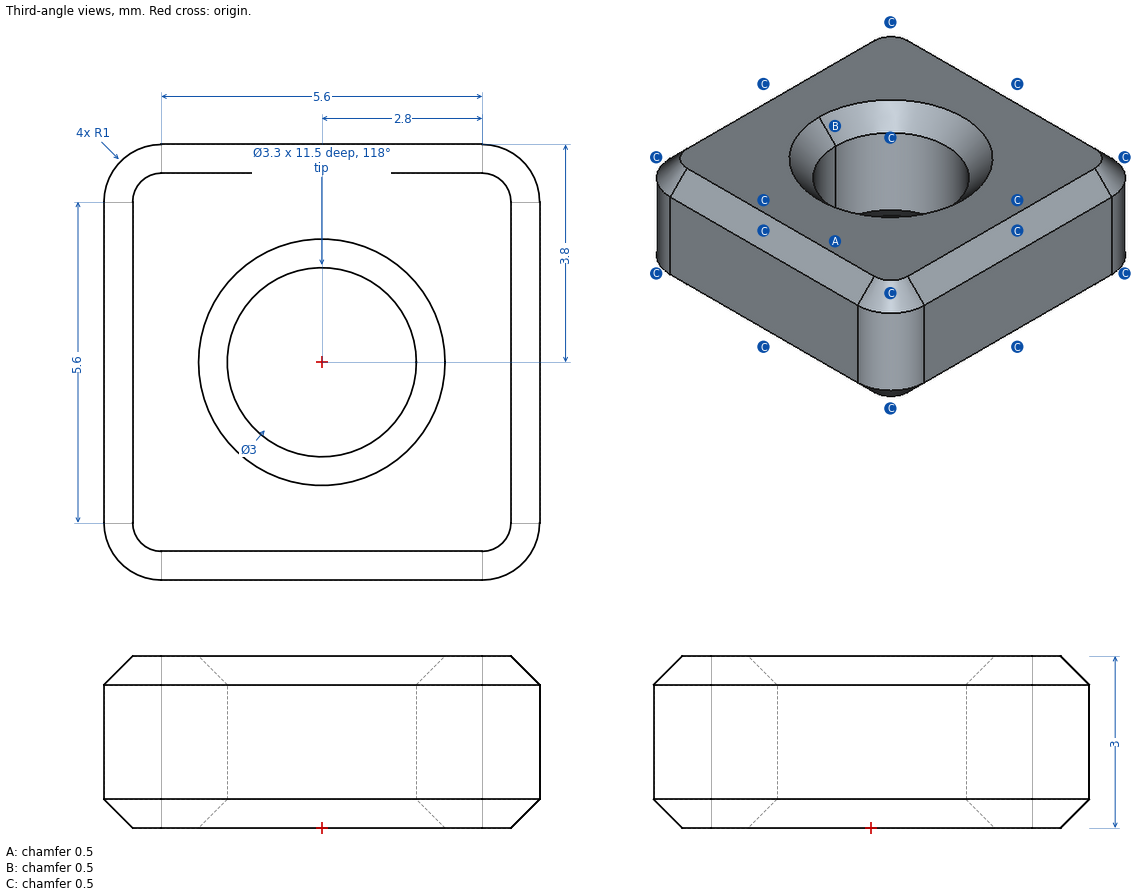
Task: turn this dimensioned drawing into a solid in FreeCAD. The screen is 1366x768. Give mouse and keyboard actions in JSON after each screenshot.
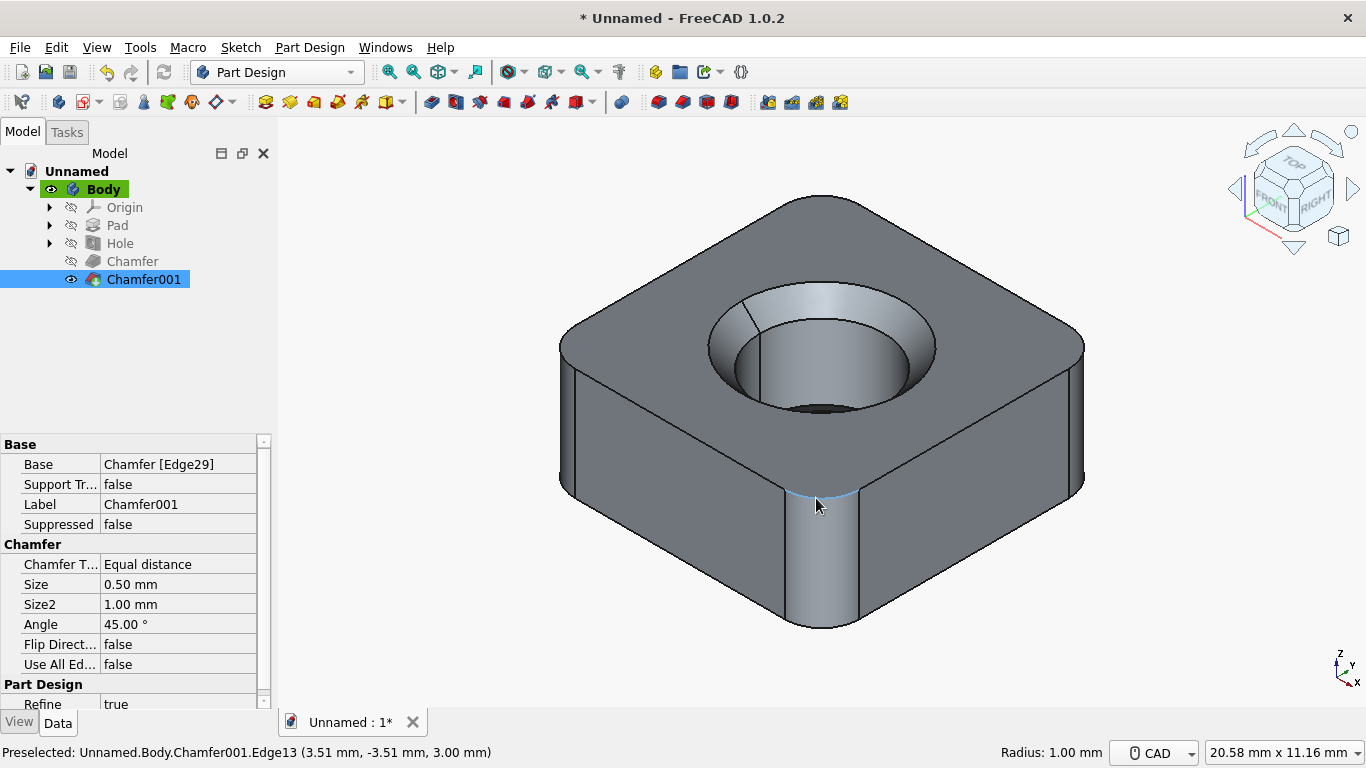
{"action": "left_click", "coordinate": [562, 485], "text": "ctrl"}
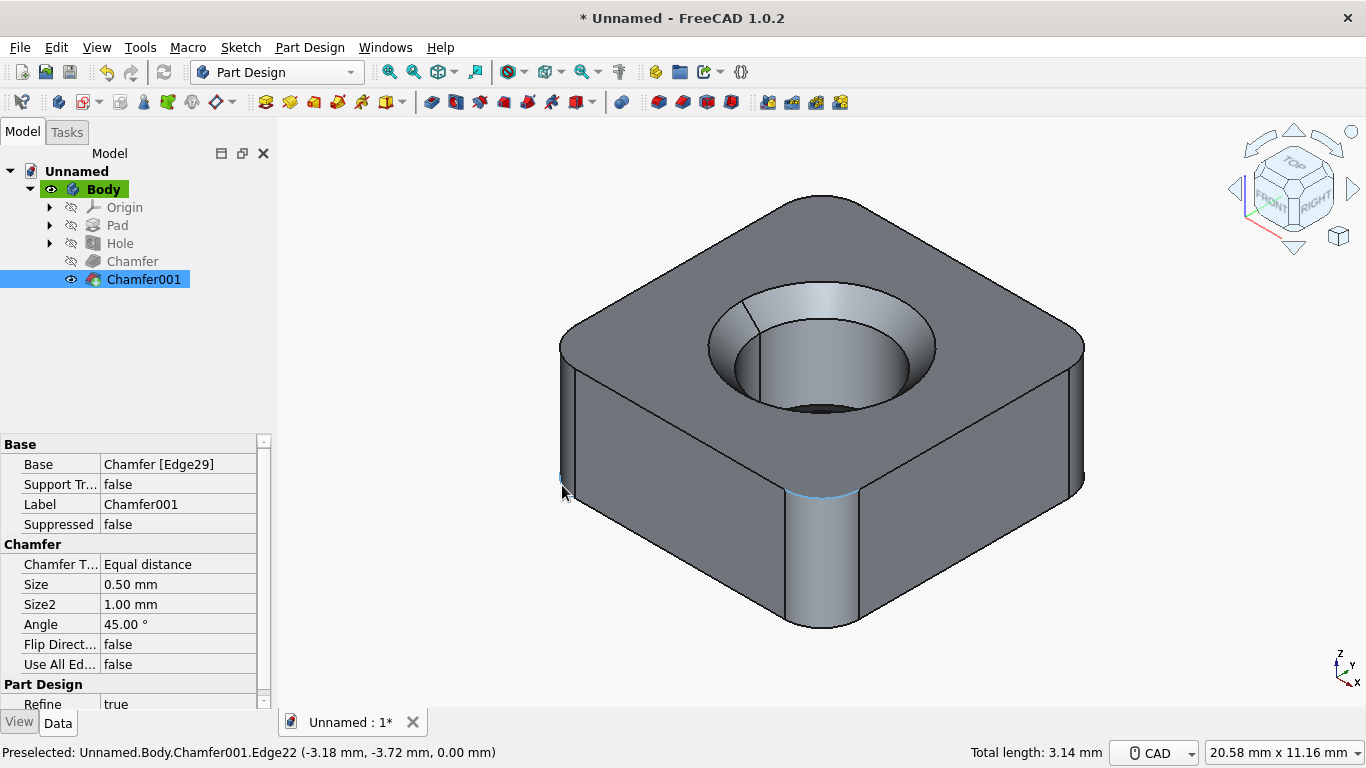
{"action": "left_click", "coordinate": [964, 428], "text": "ctrl"}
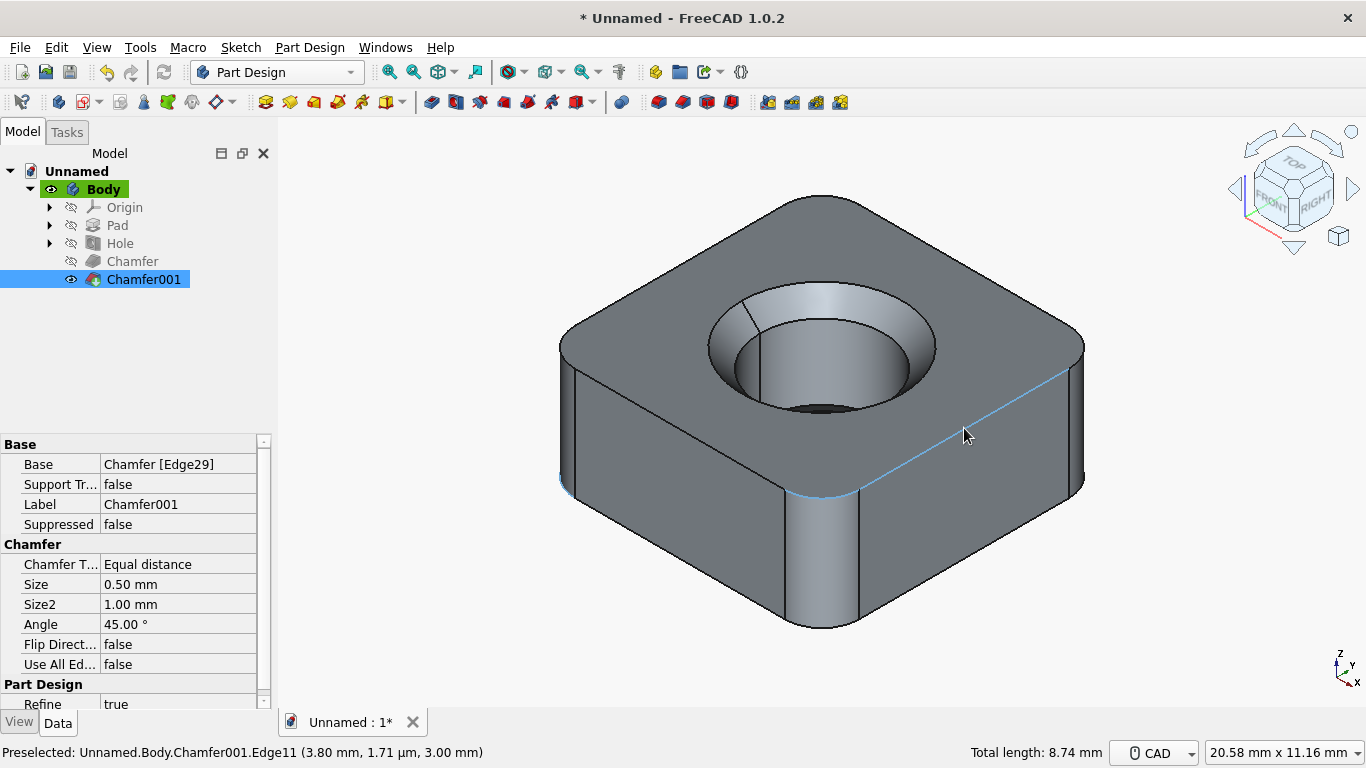
{"action": "left_click", "coordinate": [1084, 346], "text": "ctrl"}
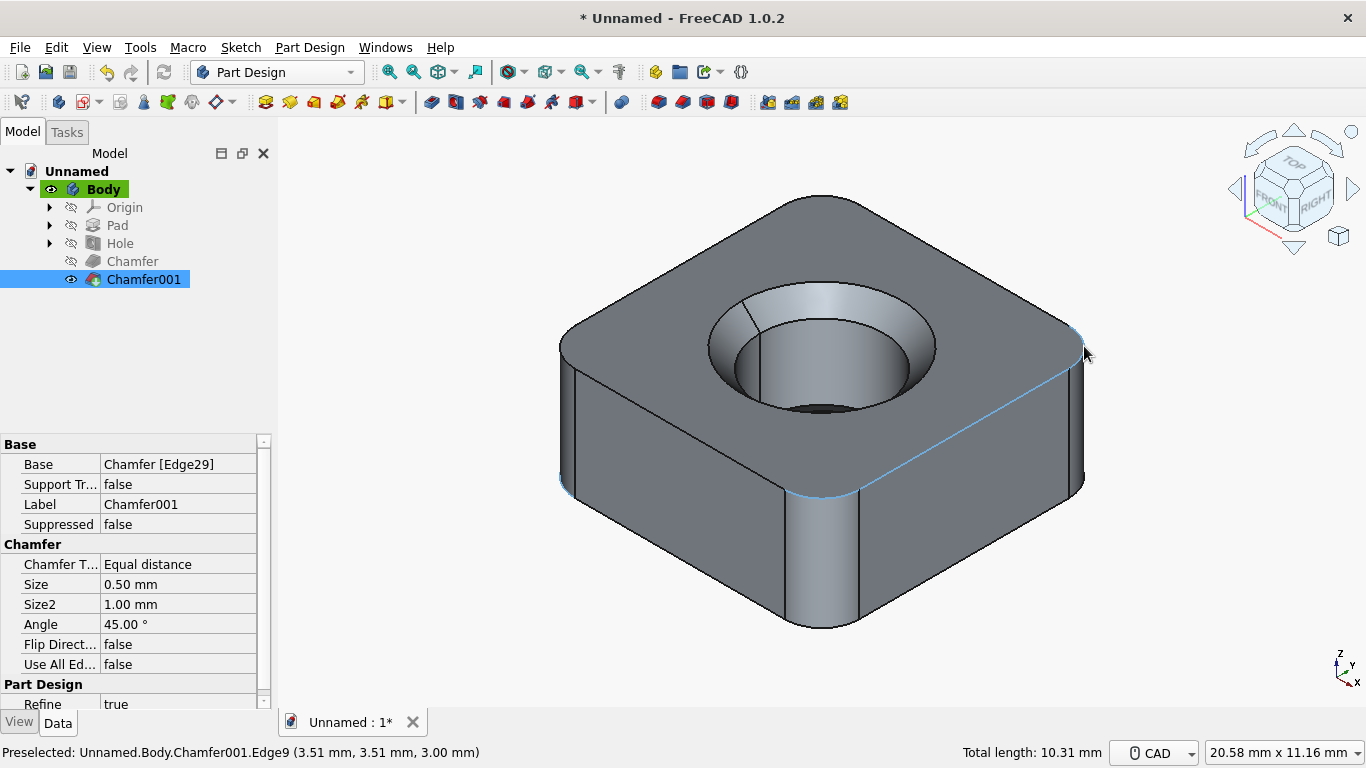
{"action": "left_click", "coordinate": [560, 346], "text": "ctrl"}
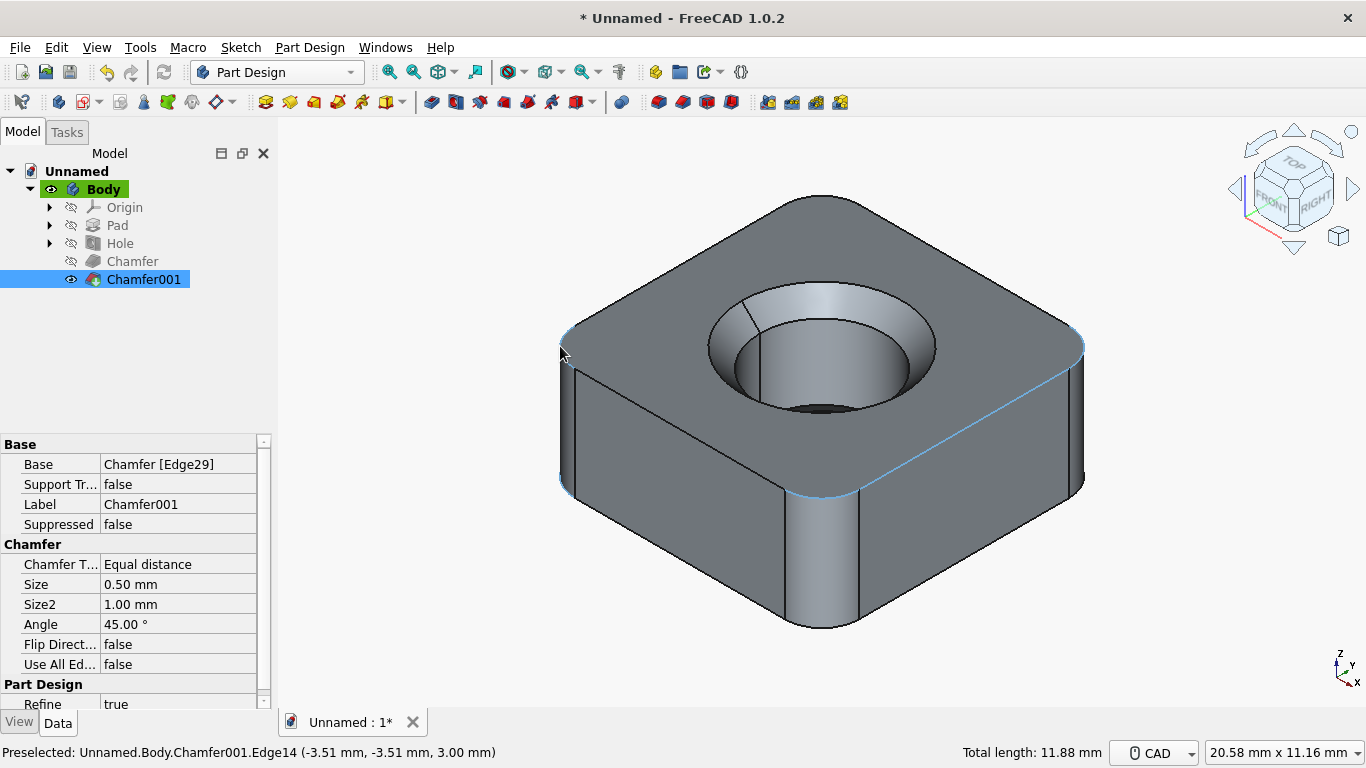
{"action": "left_click", "coordinate": [680, 428], "text": "ctrl"}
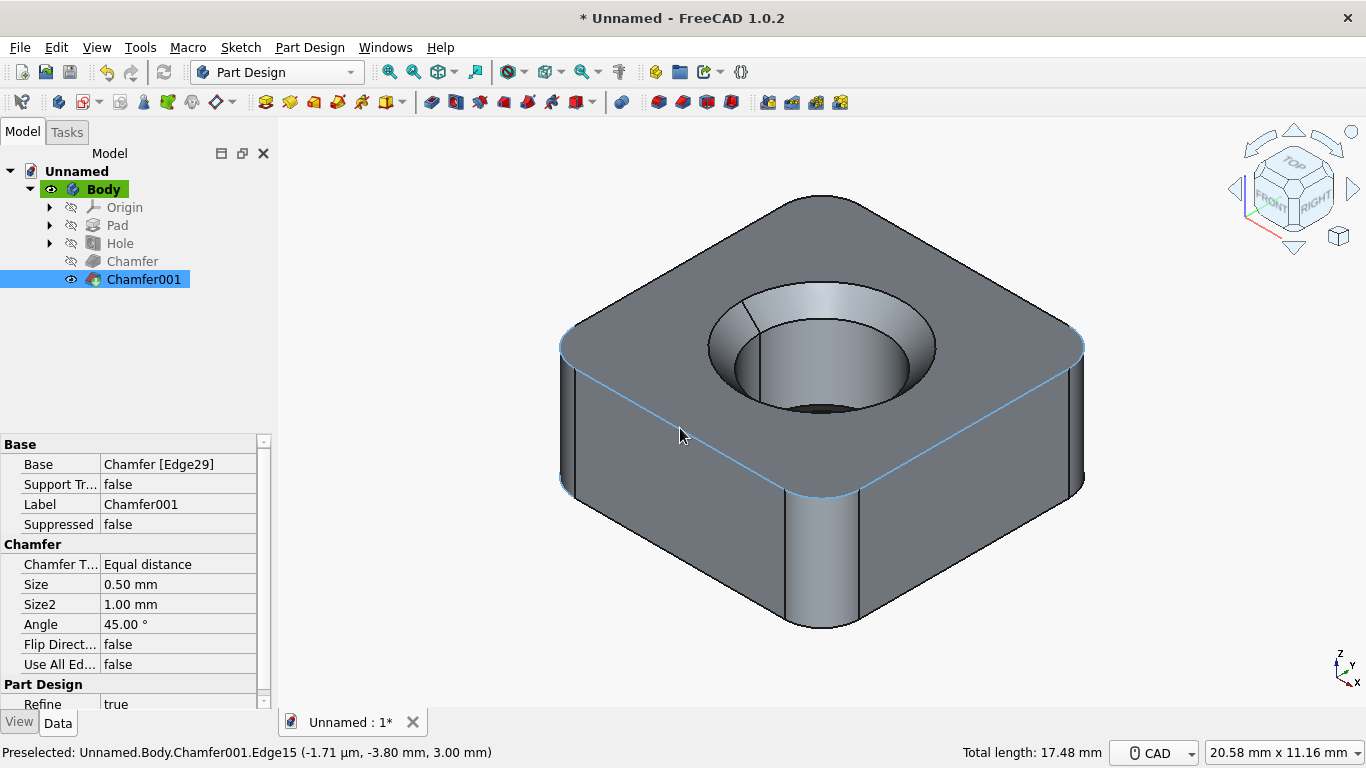
{"action": "left_click", "coordinate": [1082, 485], "text": "ctrl"}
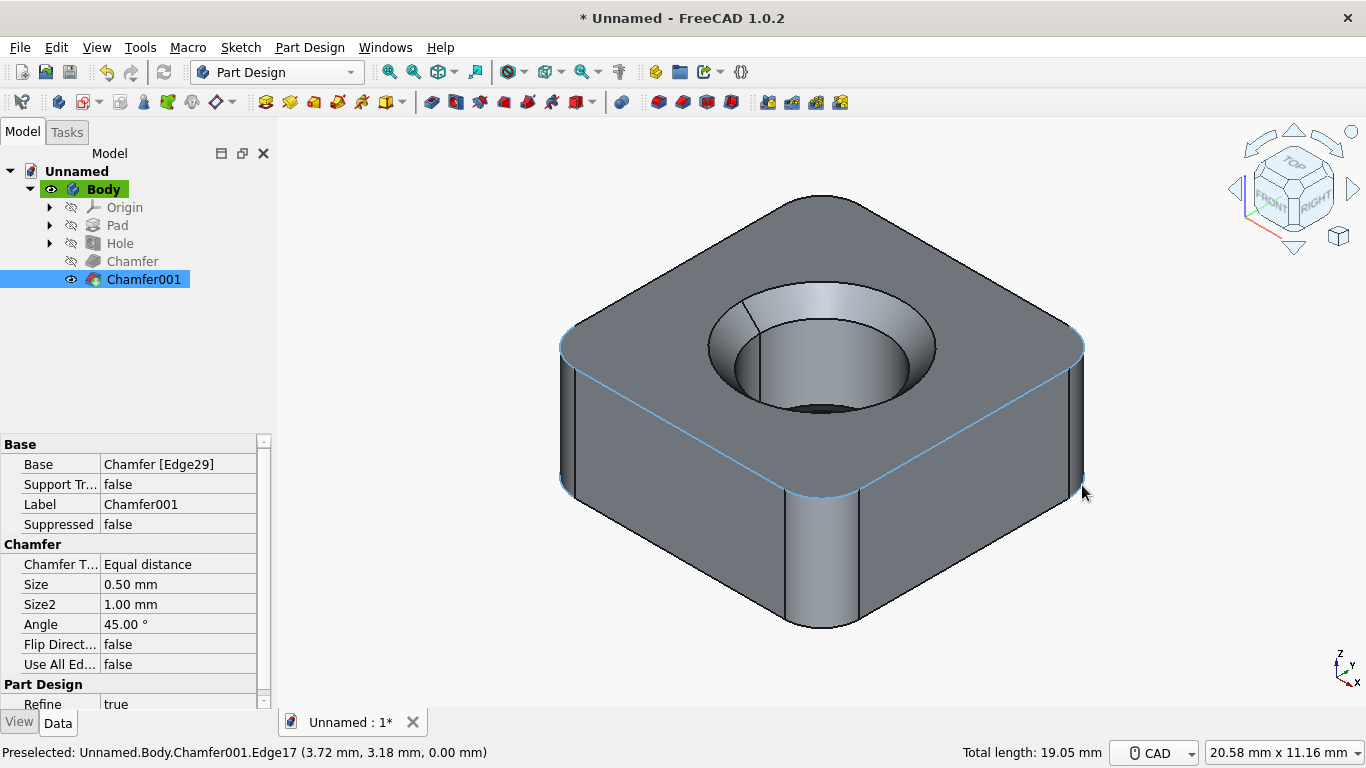
{"action": "key", "text": "2"}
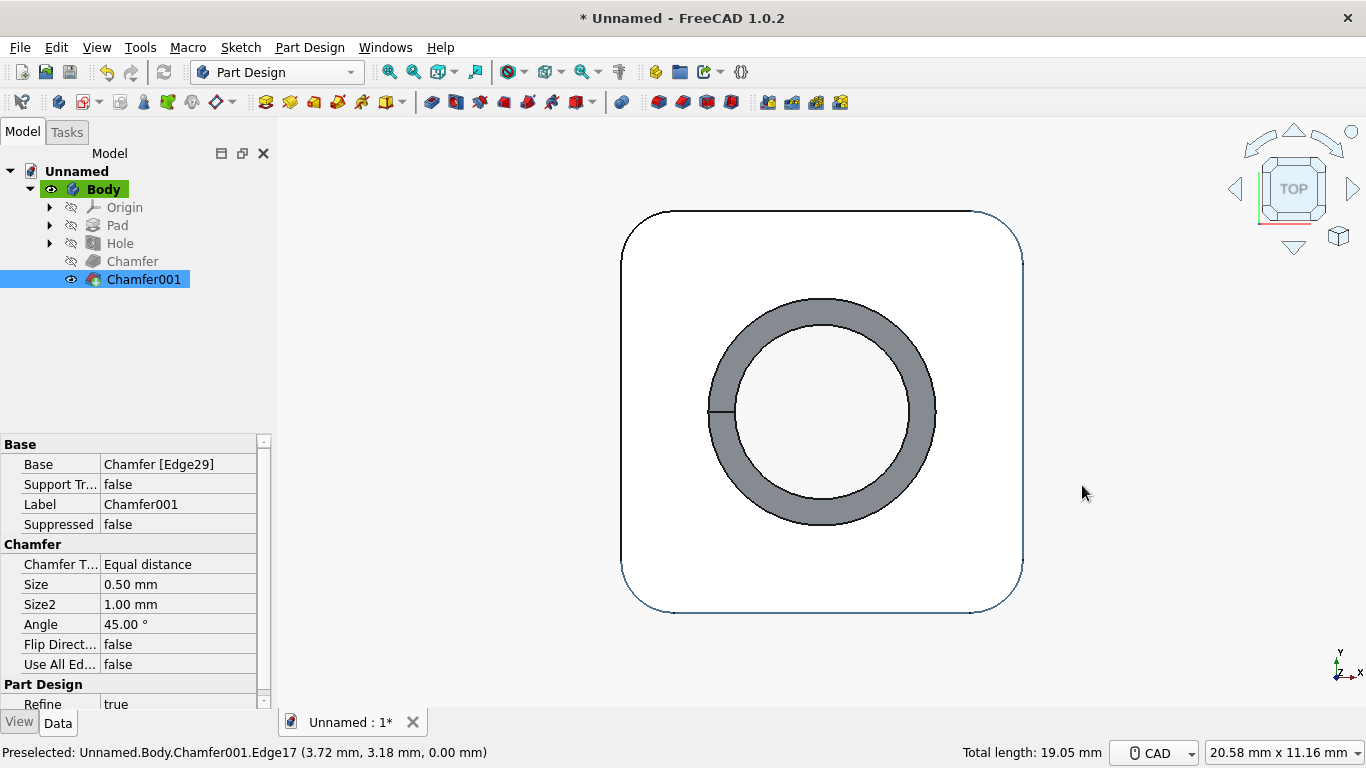
{"action": "left_click", "coordinate": [822, 210], "text": "ctrl"}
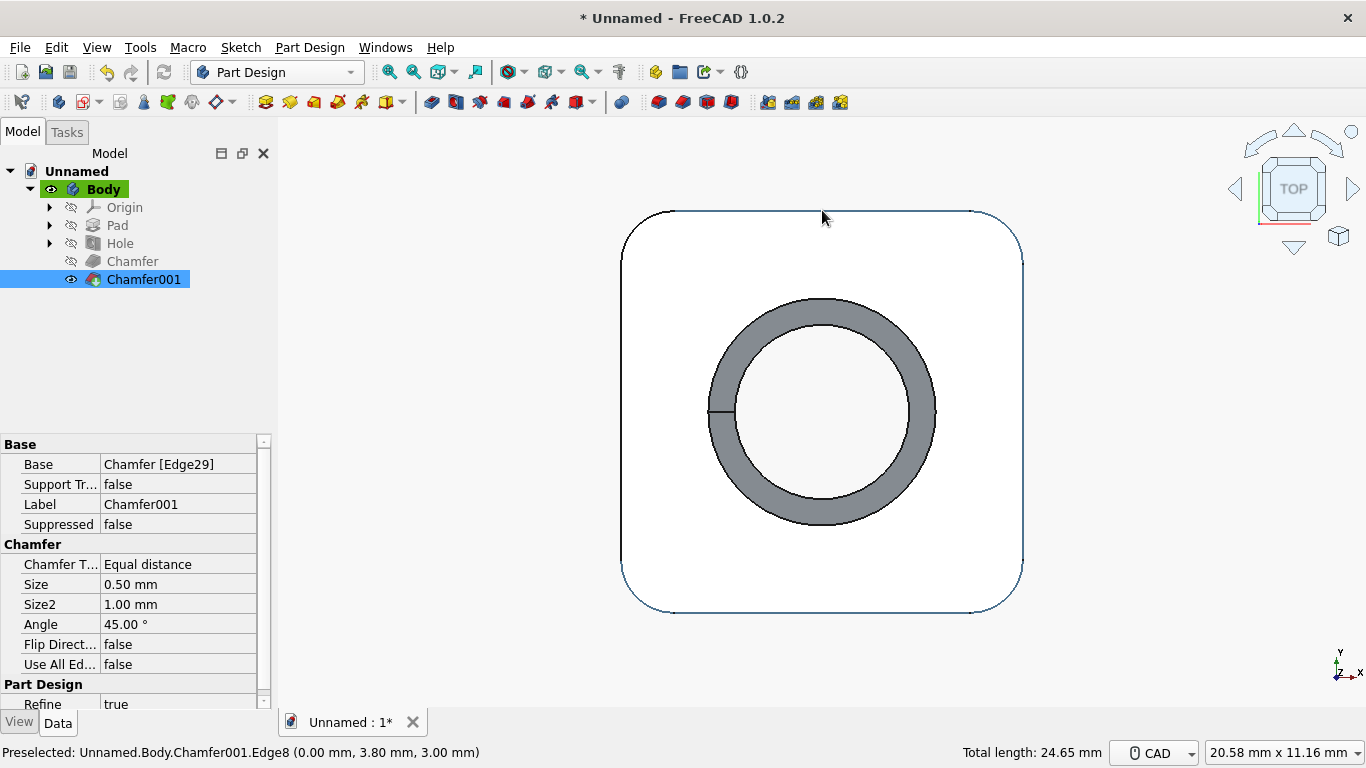
{"action": "left_click", "coordinate": [637, 226], "text": "ctrl"}